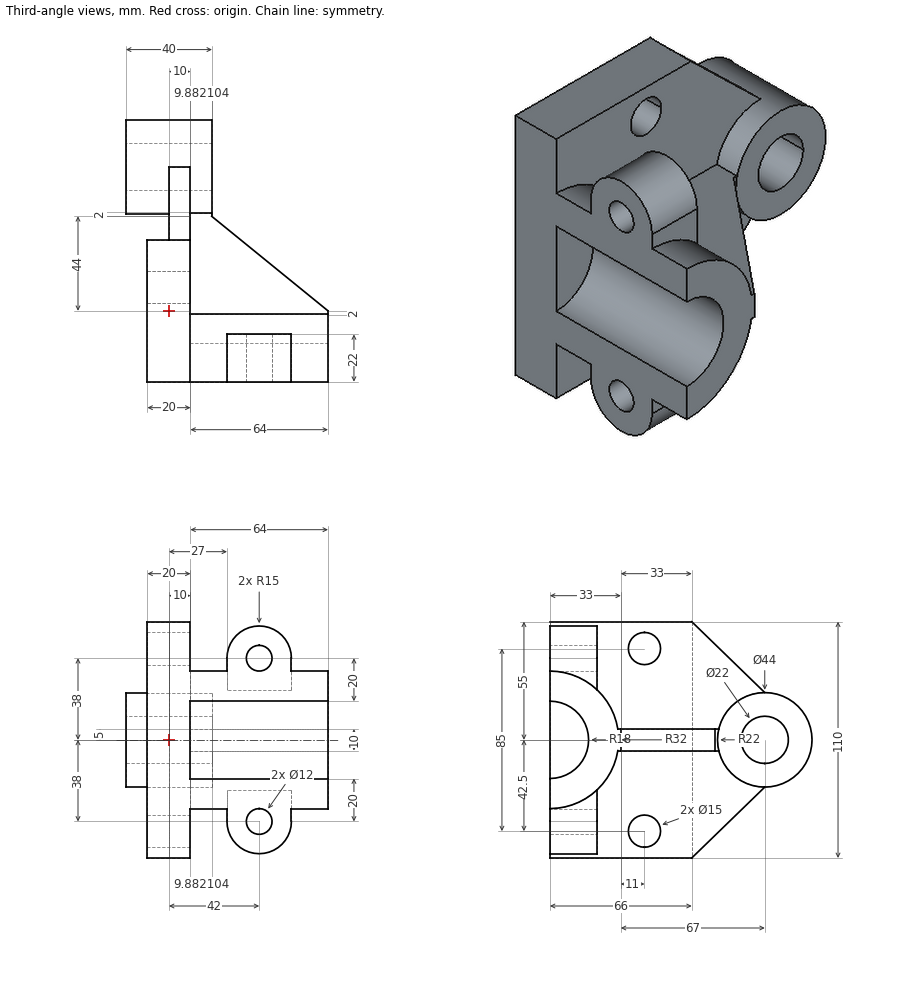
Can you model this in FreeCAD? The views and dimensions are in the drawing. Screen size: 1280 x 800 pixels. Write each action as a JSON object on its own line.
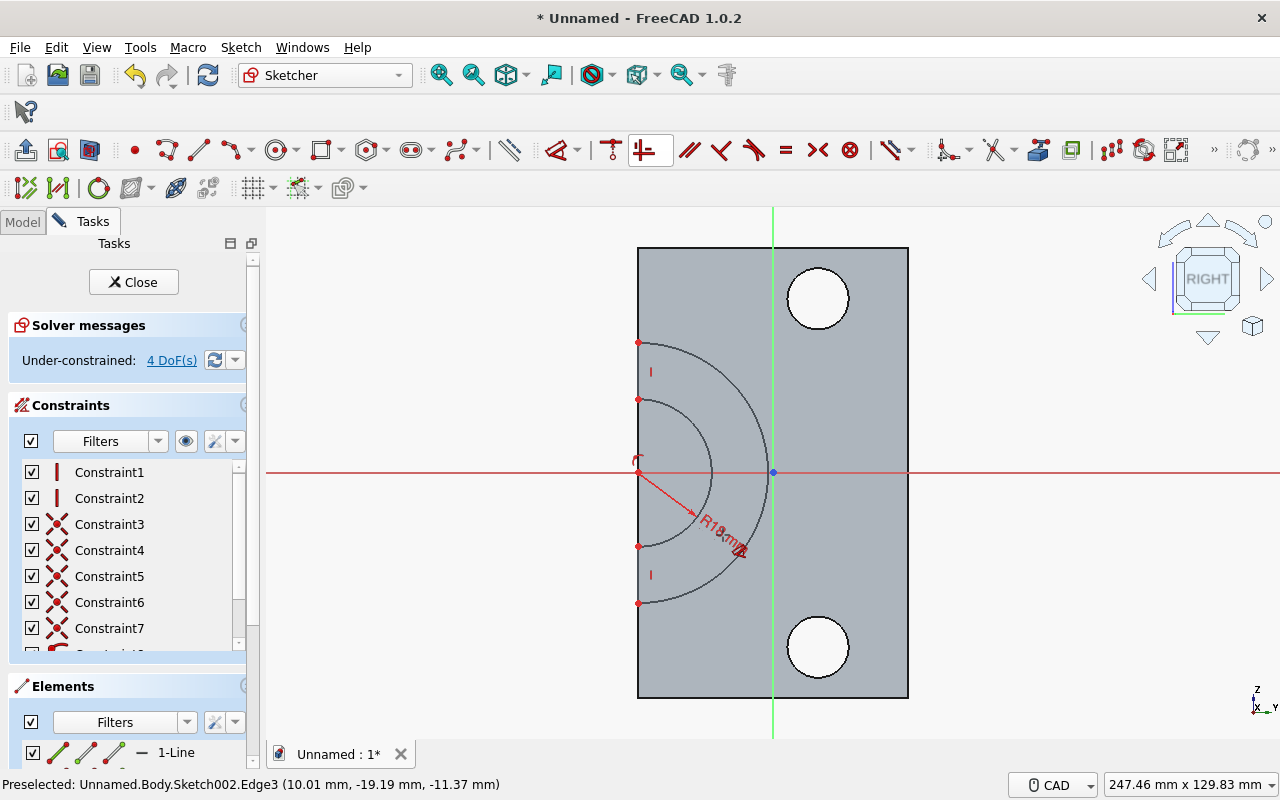
{"action": "left_click", "coordinate": [743, 549]}
{"action": "left_click", "coordinate": [707, 619]}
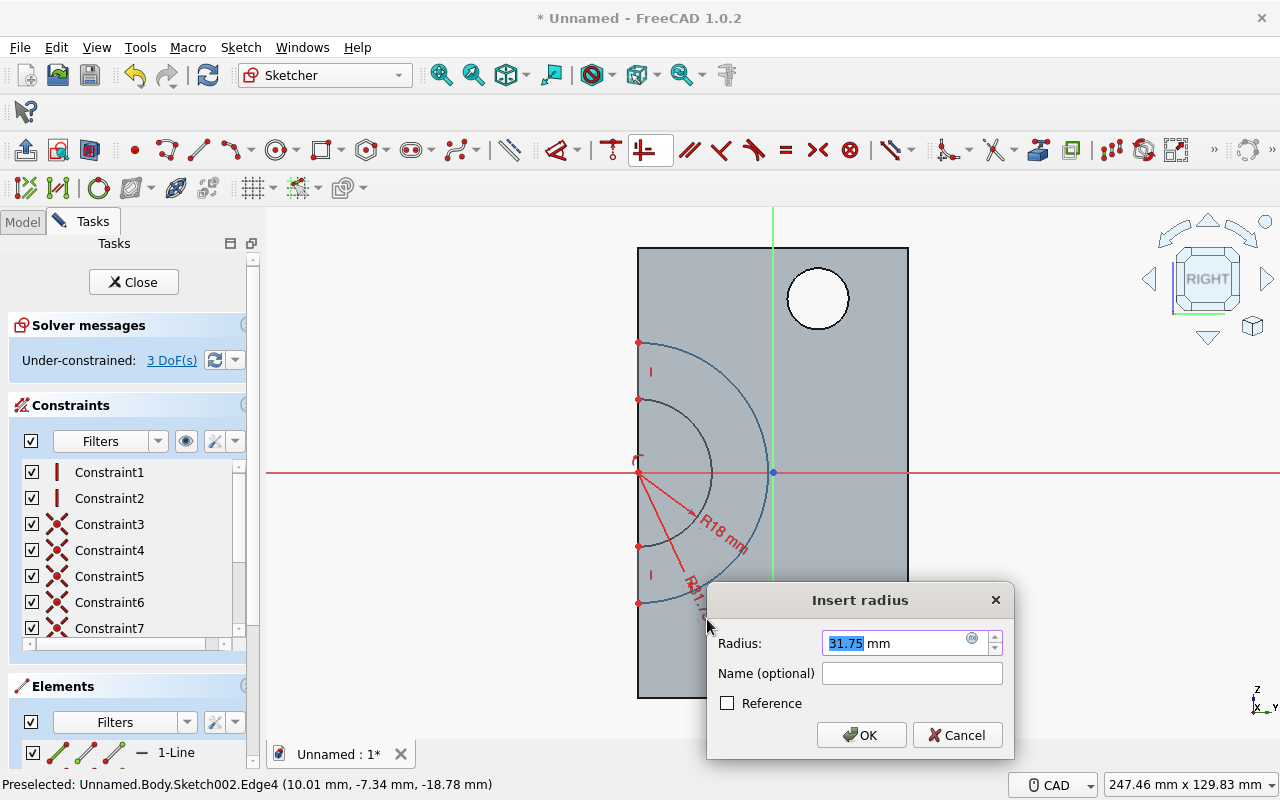
{"action": "type", "text": "32"}
{"action": "key", "text": "Return"}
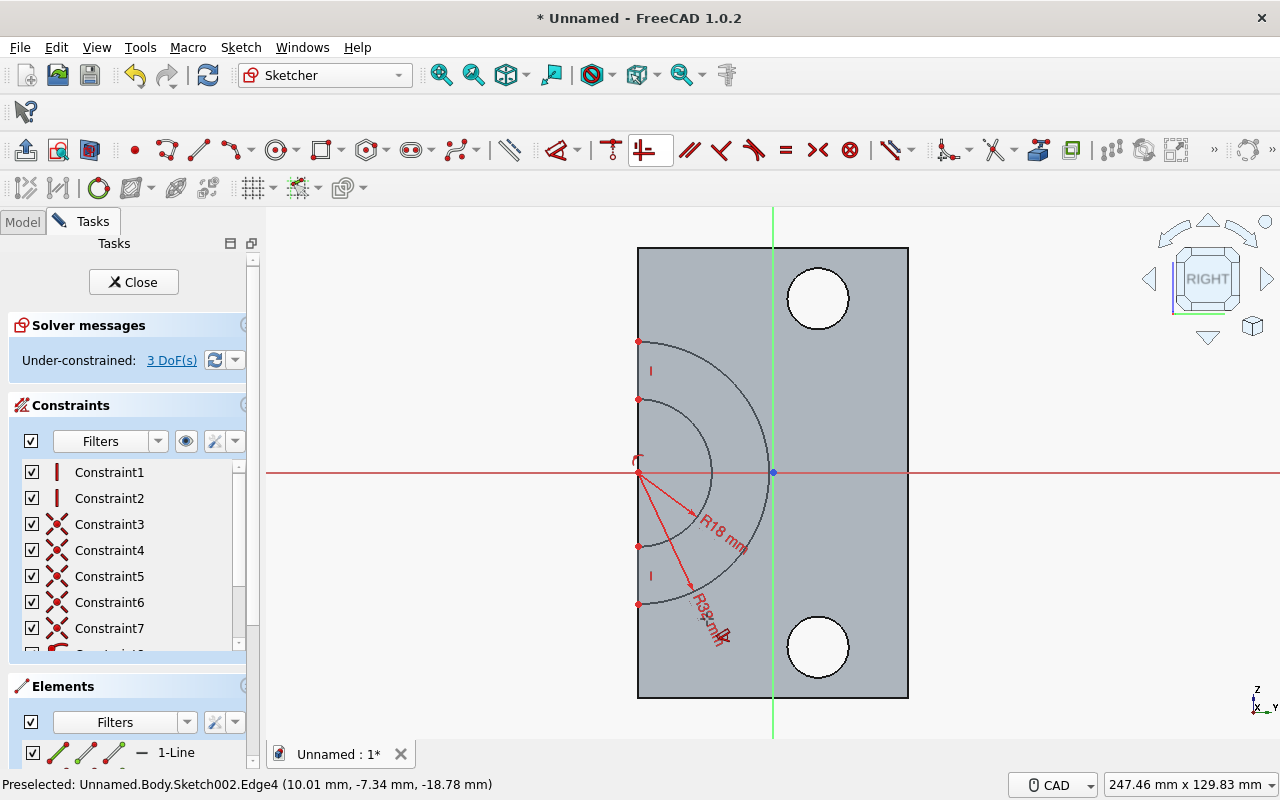
{"action": "left_click", "coordinate": [638, 342]}
{"action": "left_click", "coordinate": [705, 308]}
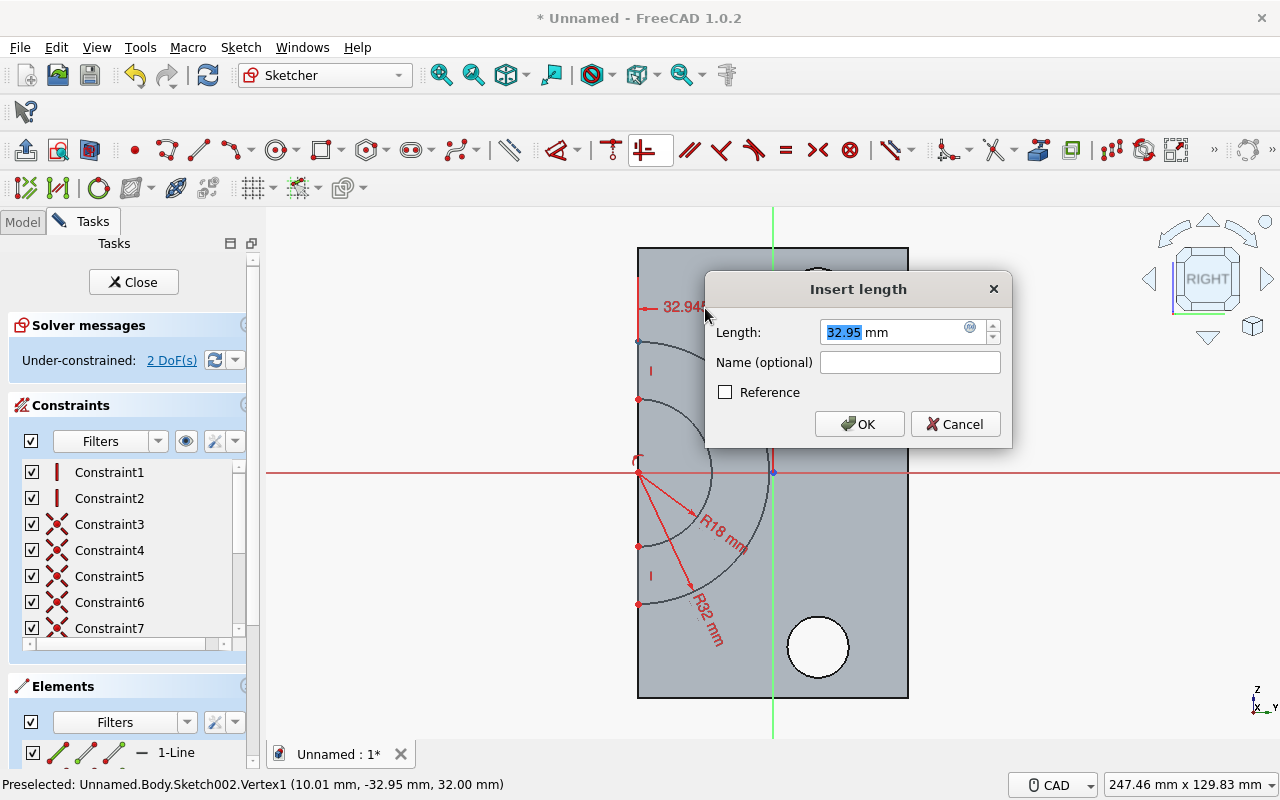
{"action": "type", "text": "33"}
{"action": "key", "text": "Return"}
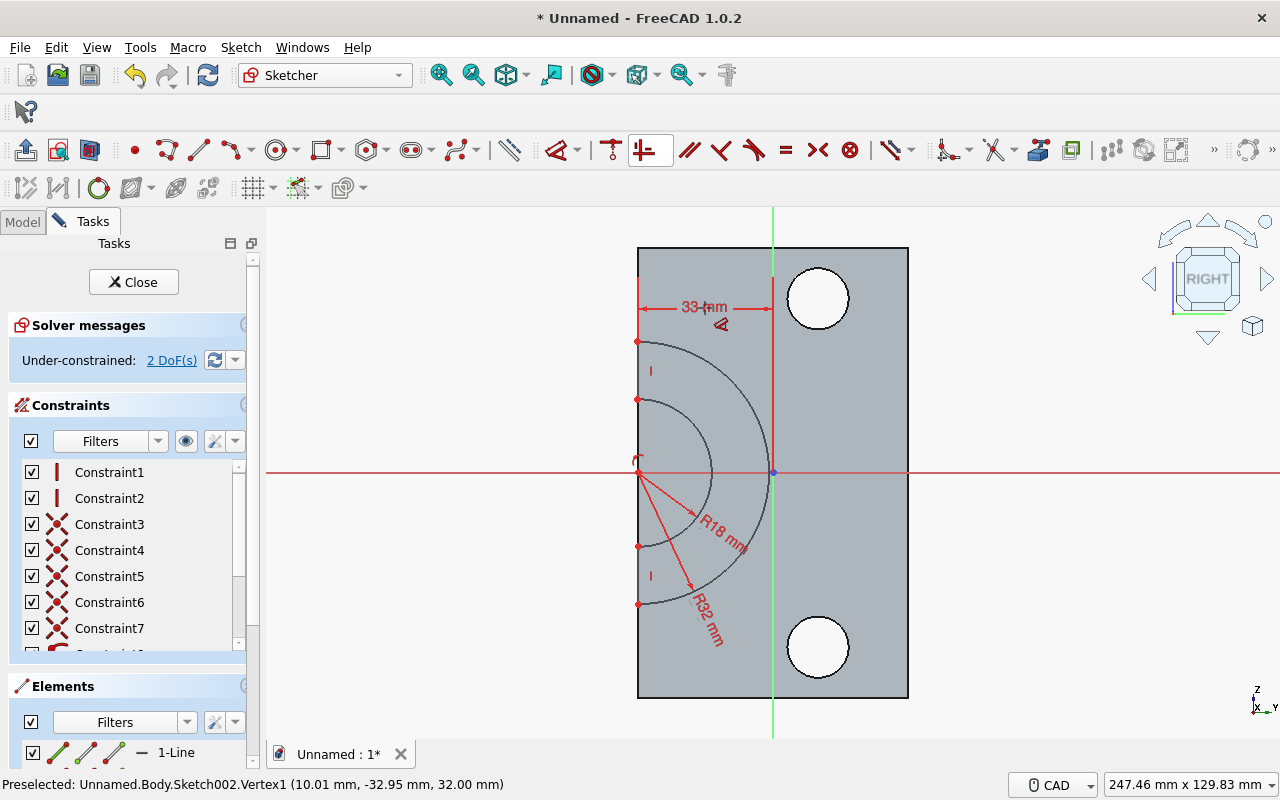
{"action": "left_click", "coordinate": [638, 547]}
{"action": "left_click", "coordinate": [674, 581]}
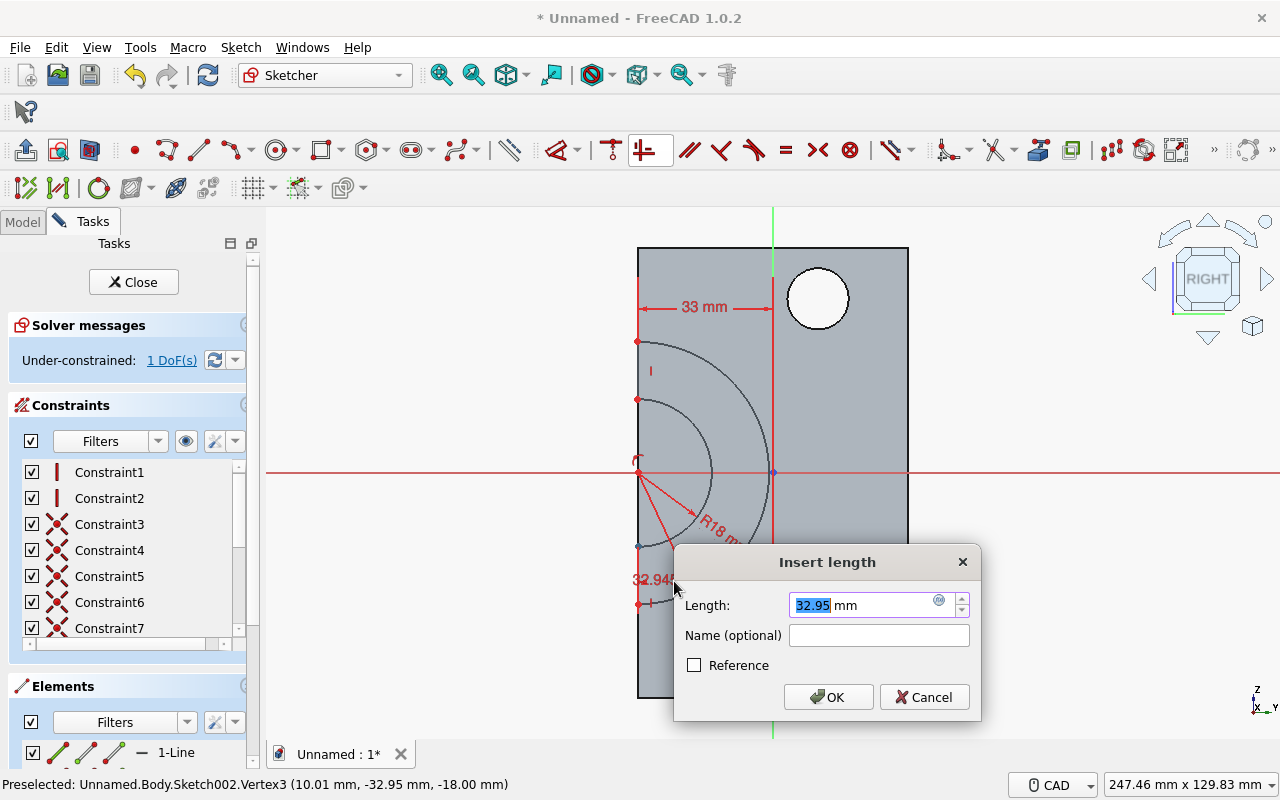
{"action": "type", "text": "33"}
{"action": "key", "text": "Return"}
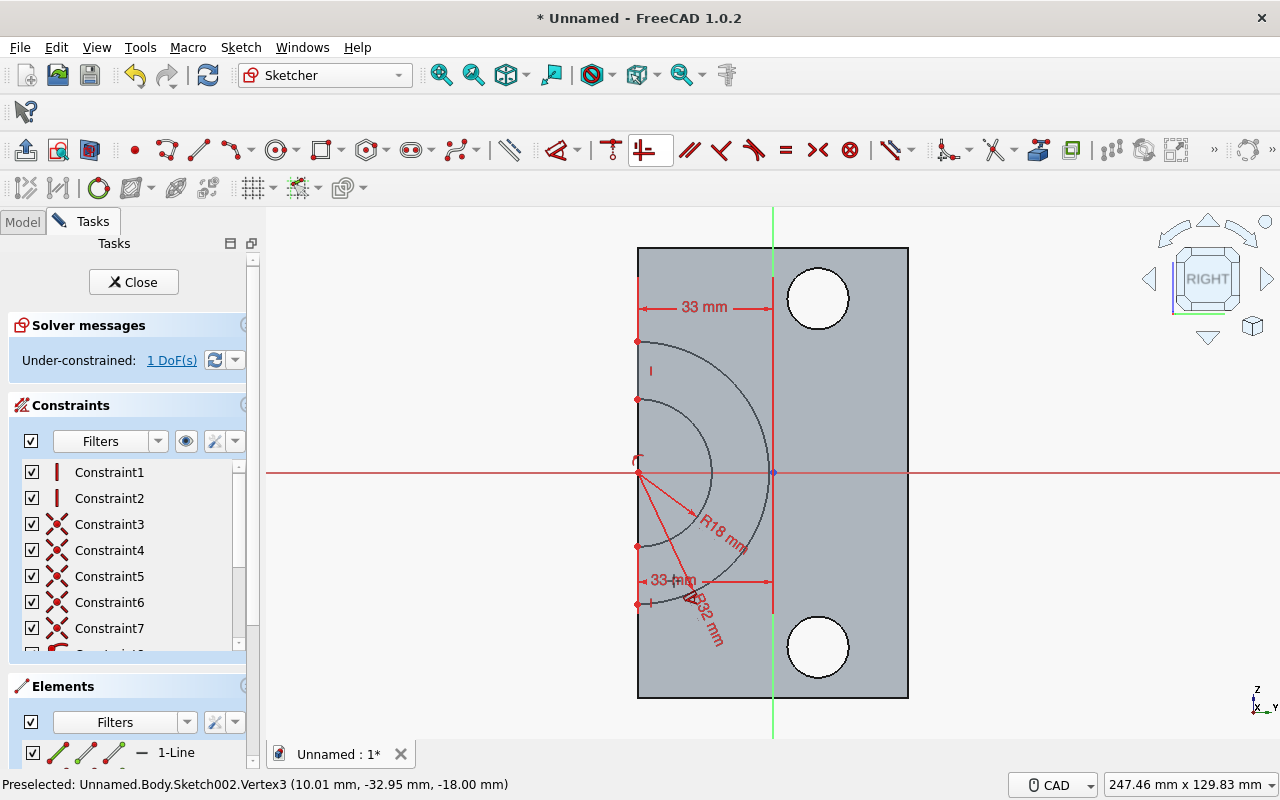
{"action": "left_click", "coordinate": [638, 473]}
{"action": "left_click", "coordinate": [674, 507]}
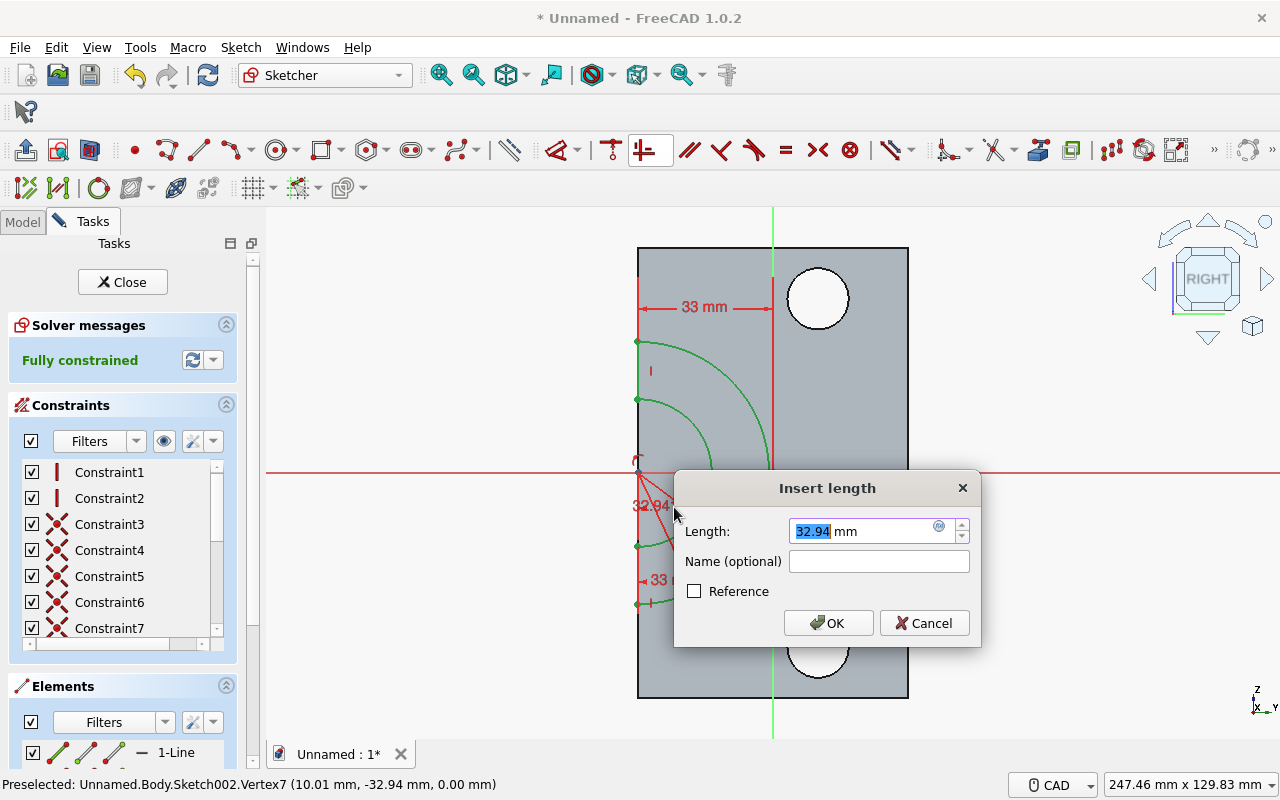
{"action": "type", "text": "33"}
{"action": "key", "text": "Return"}
{"action": "key", "text": "Escape"}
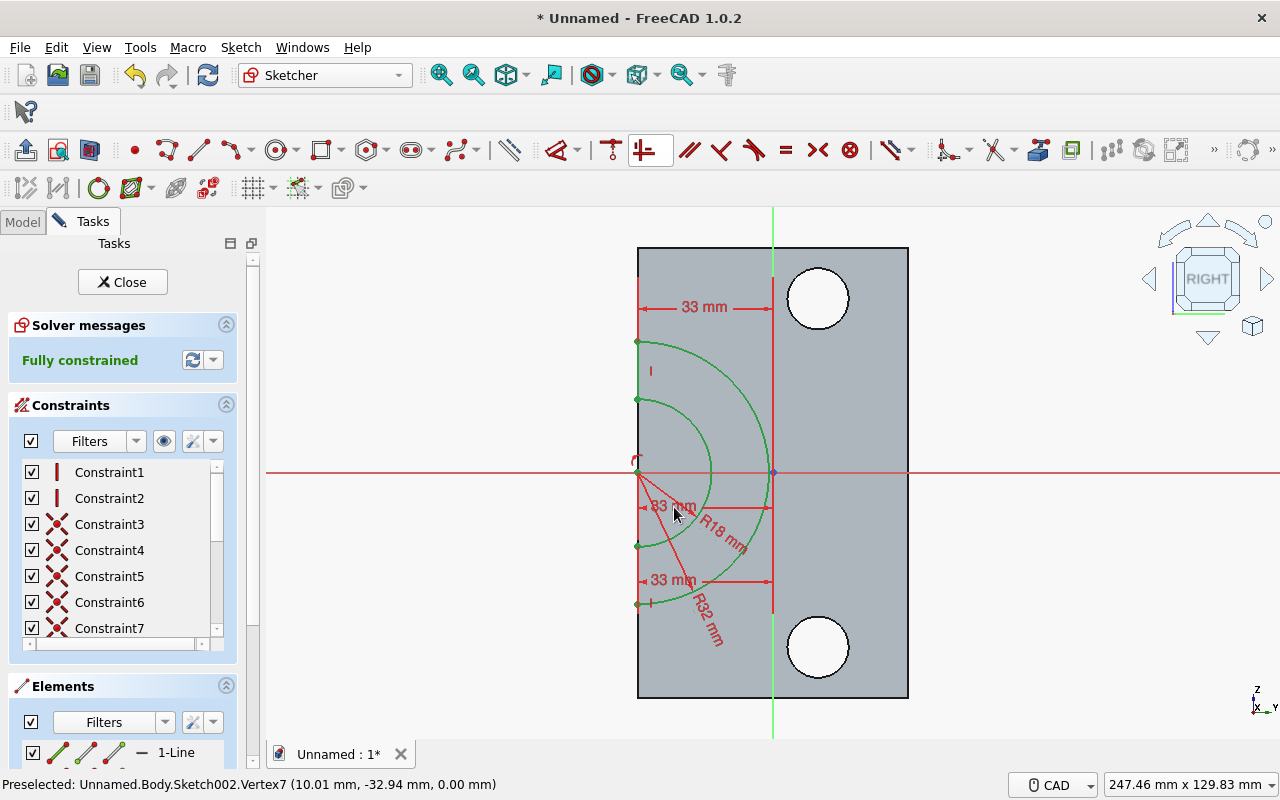
{"action": "left_click", "coordinate": [123, 282]}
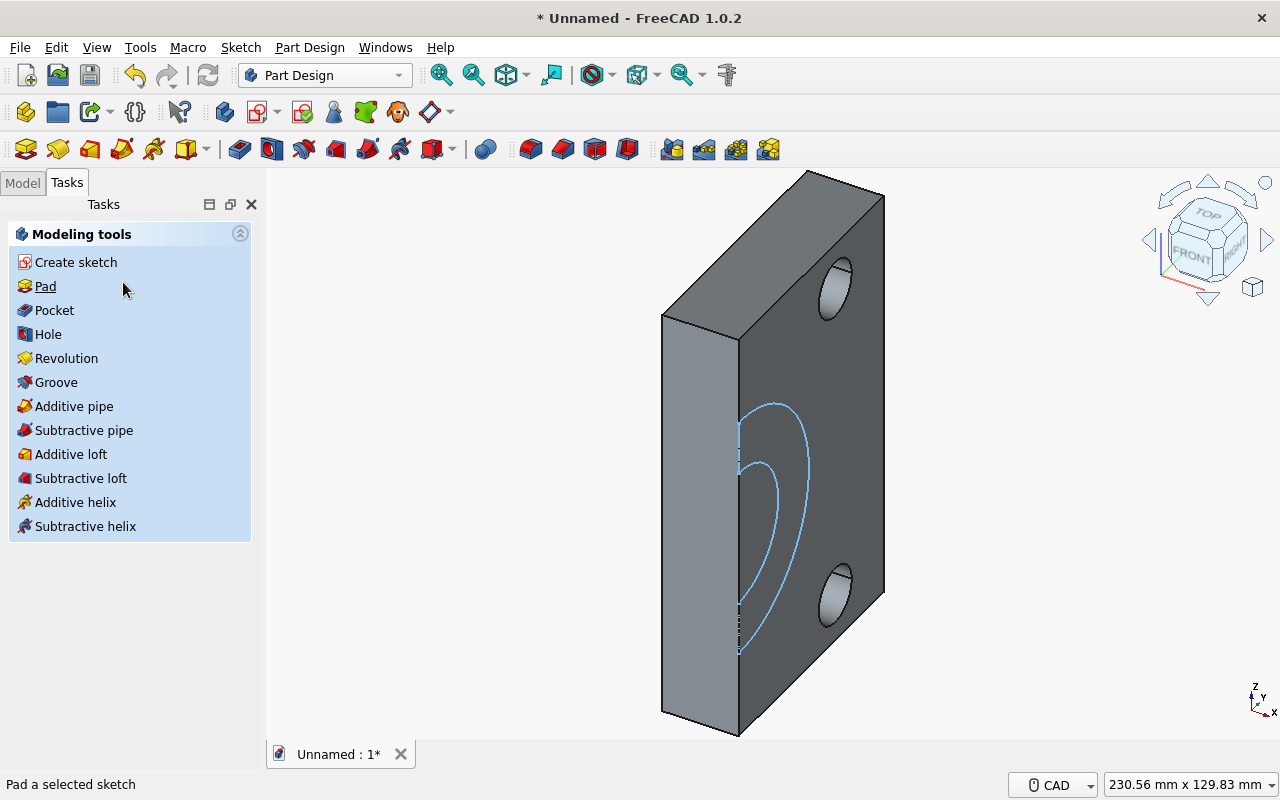
{"action": "left_click", "coordinate": [26, 150]}